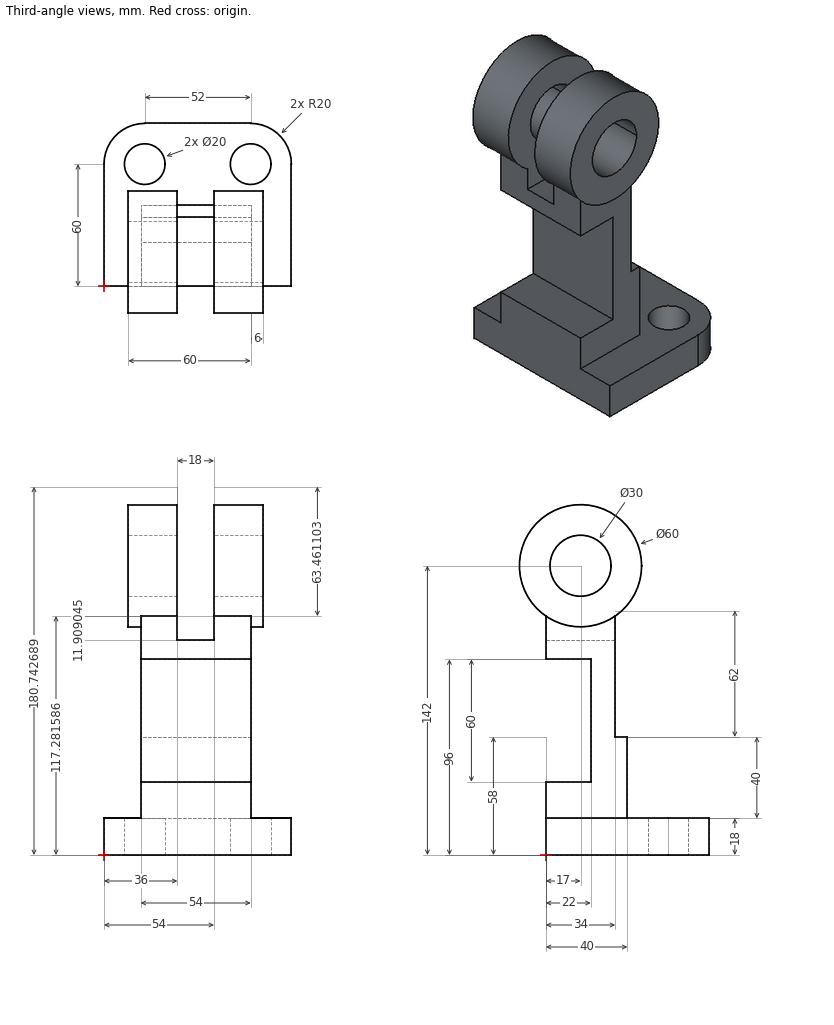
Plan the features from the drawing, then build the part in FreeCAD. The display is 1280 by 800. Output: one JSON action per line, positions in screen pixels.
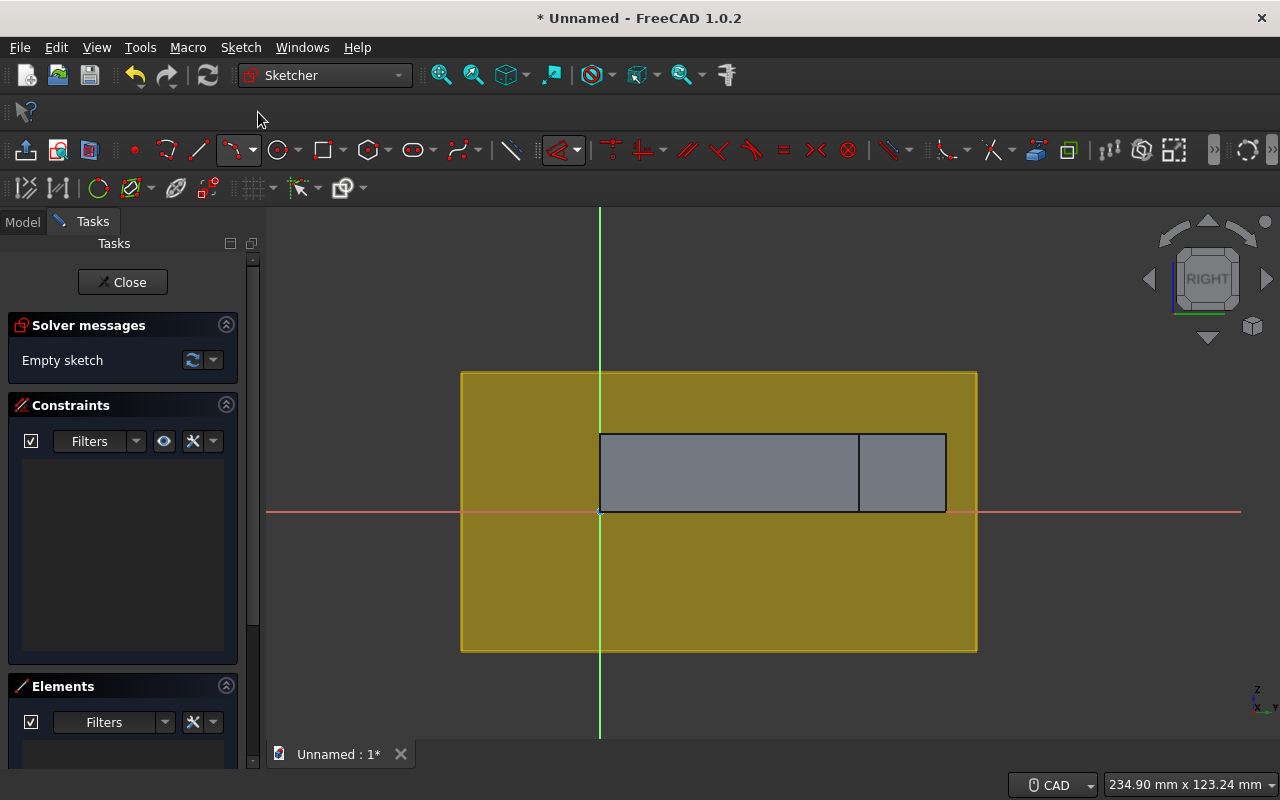
{"action": "left_click", "coordinate": [90, 150]}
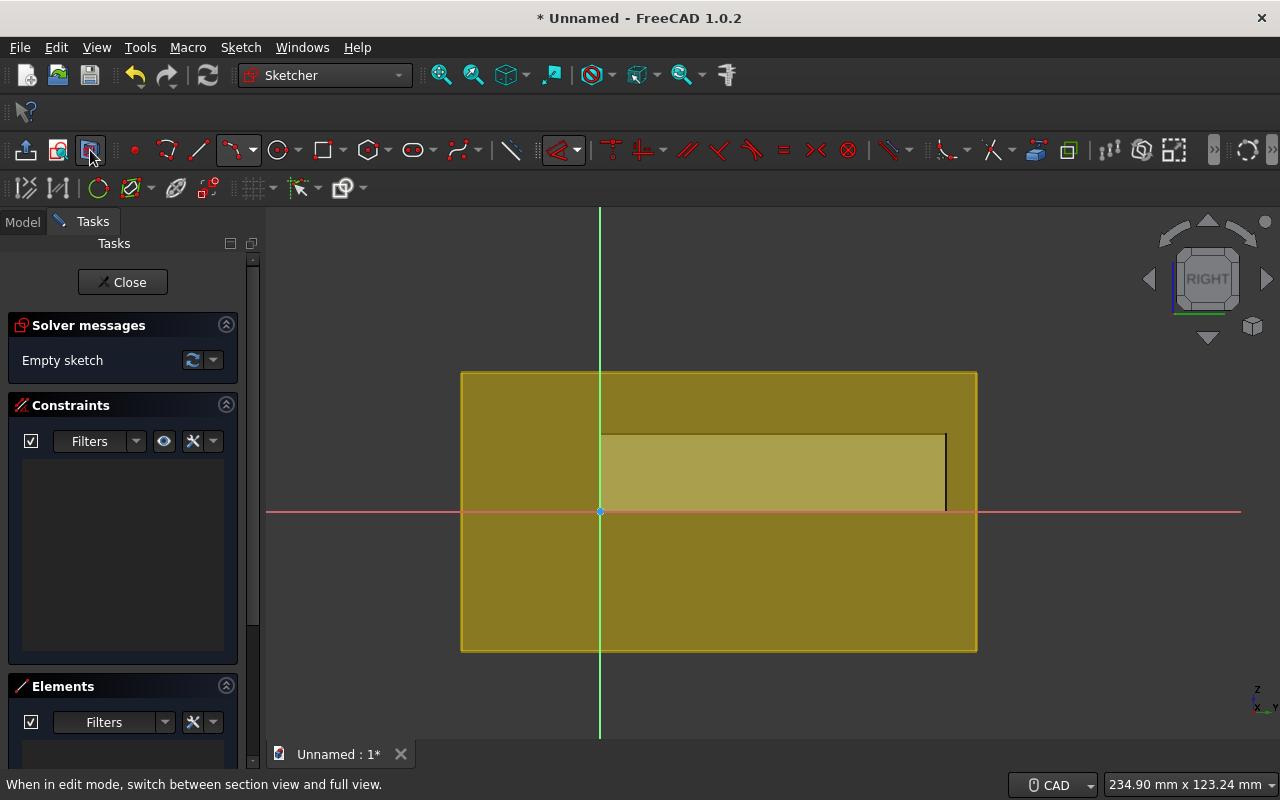
{"action": "left_click", "coordinate": [324, 150]}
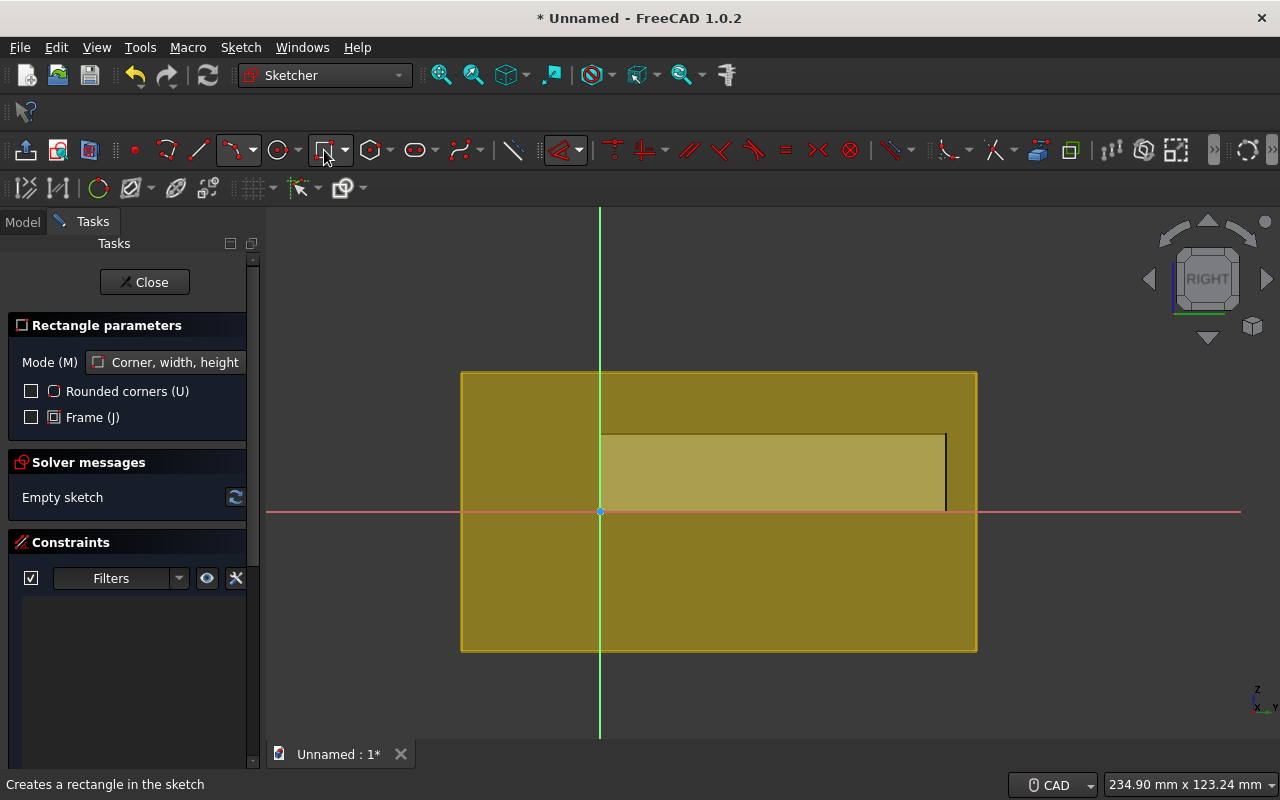
{"action": "left_click", "coordinate": [600, 261]}
{"action": "mouse_move", "coordinate": [773, 434]}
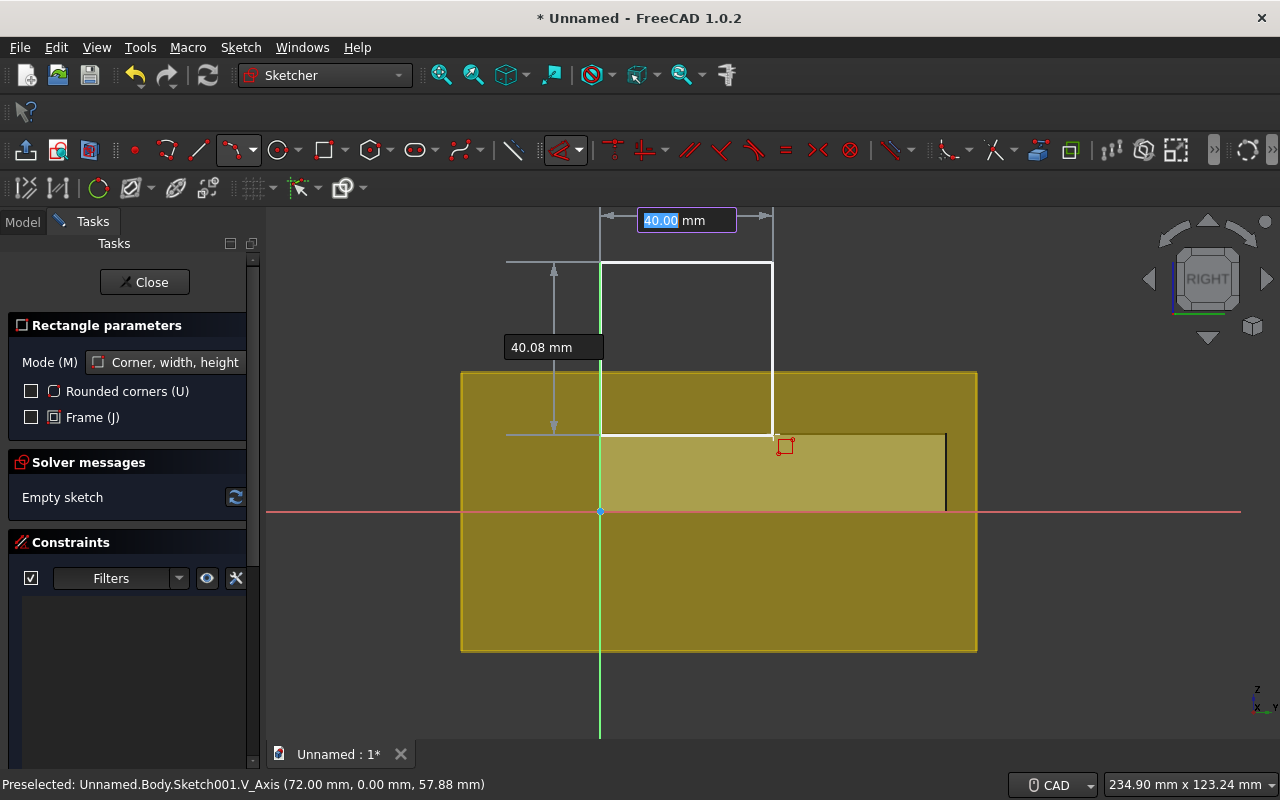
{"action": "type", "text": "40"}
{"action": "key", "text": "Tab"}
{"action": "type", "text": "40"}
{"action": "key", "text": "Return"}
{"action": "key", "text": "Escape"}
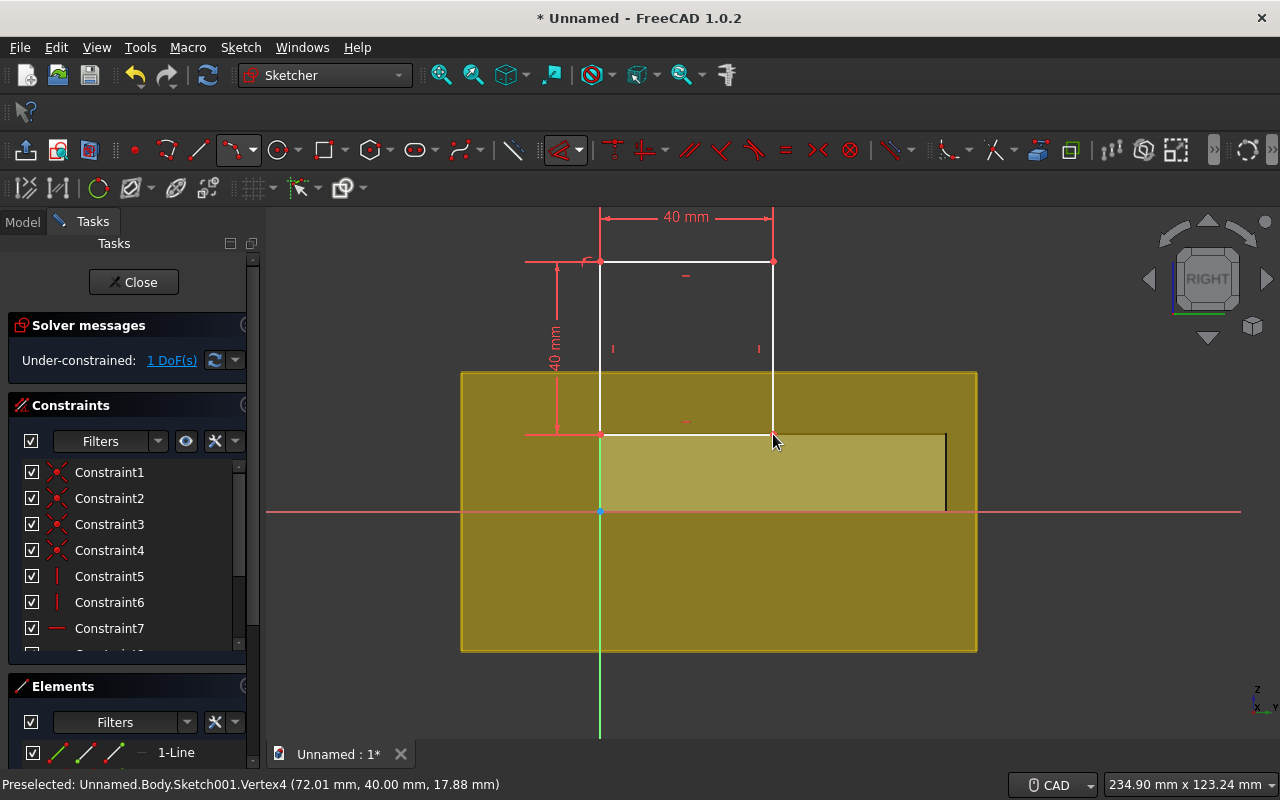
{"action": "left_click", "coordinate": [600, 262]}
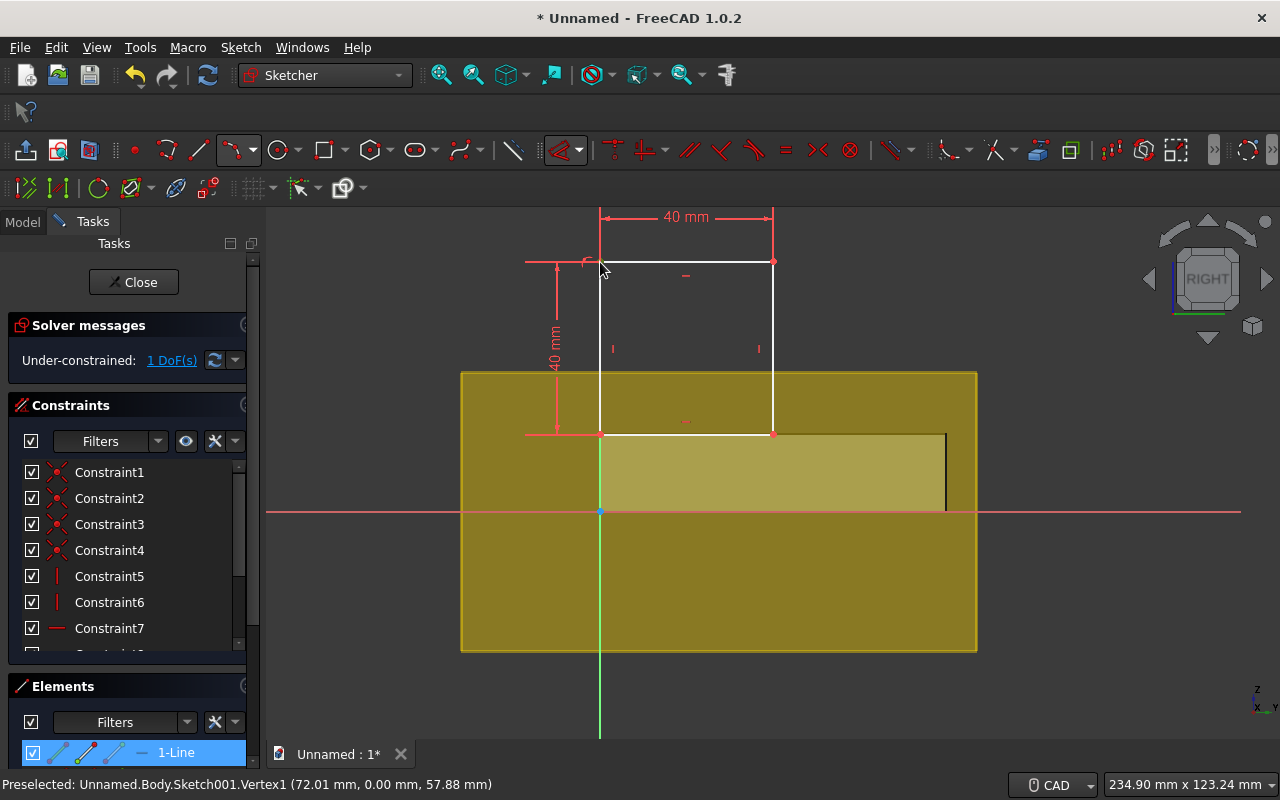
{"action": "left_click", "coordinate": [582, 150]}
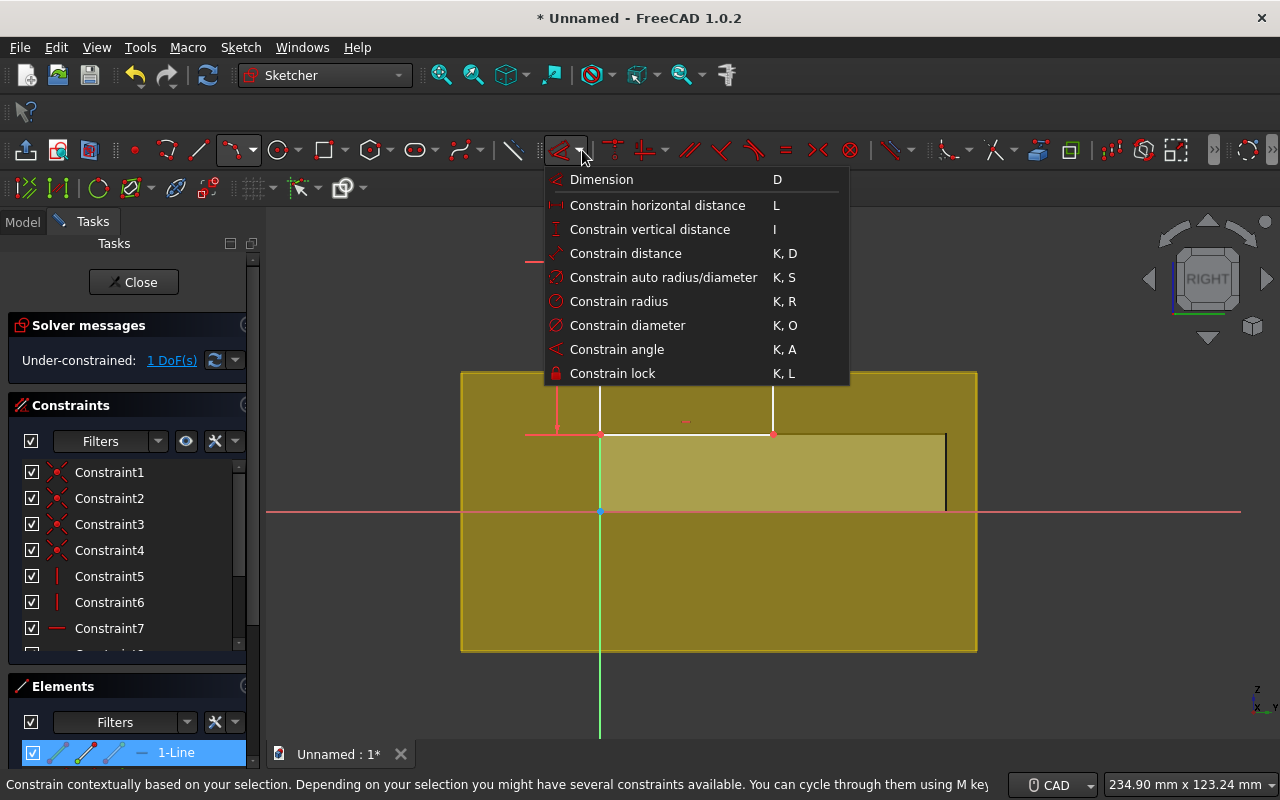
{"action": "left_click", "coordinate": [697, 229]}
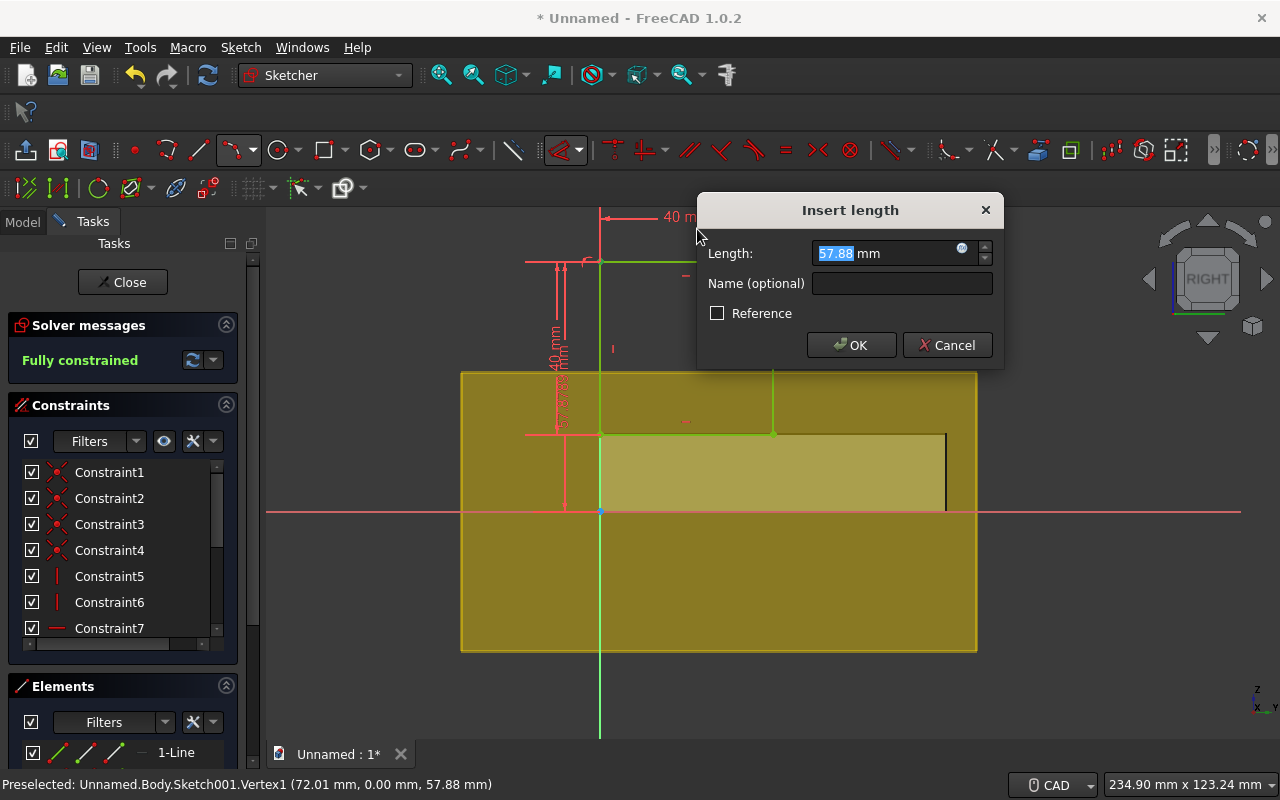
{"action": "type", "text": "58"}
{"action": "key", "text": "Return"}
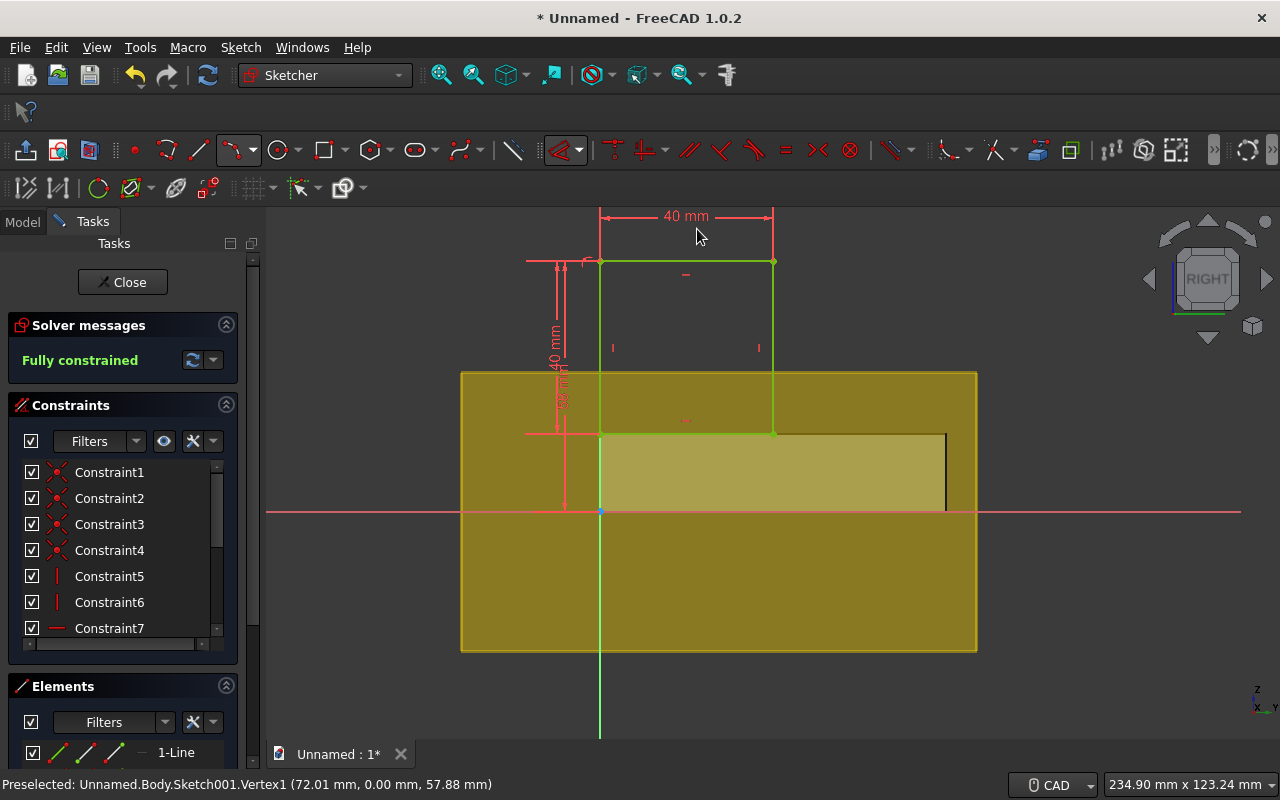
{"action": "left_click", "coordinate": [123, 282]}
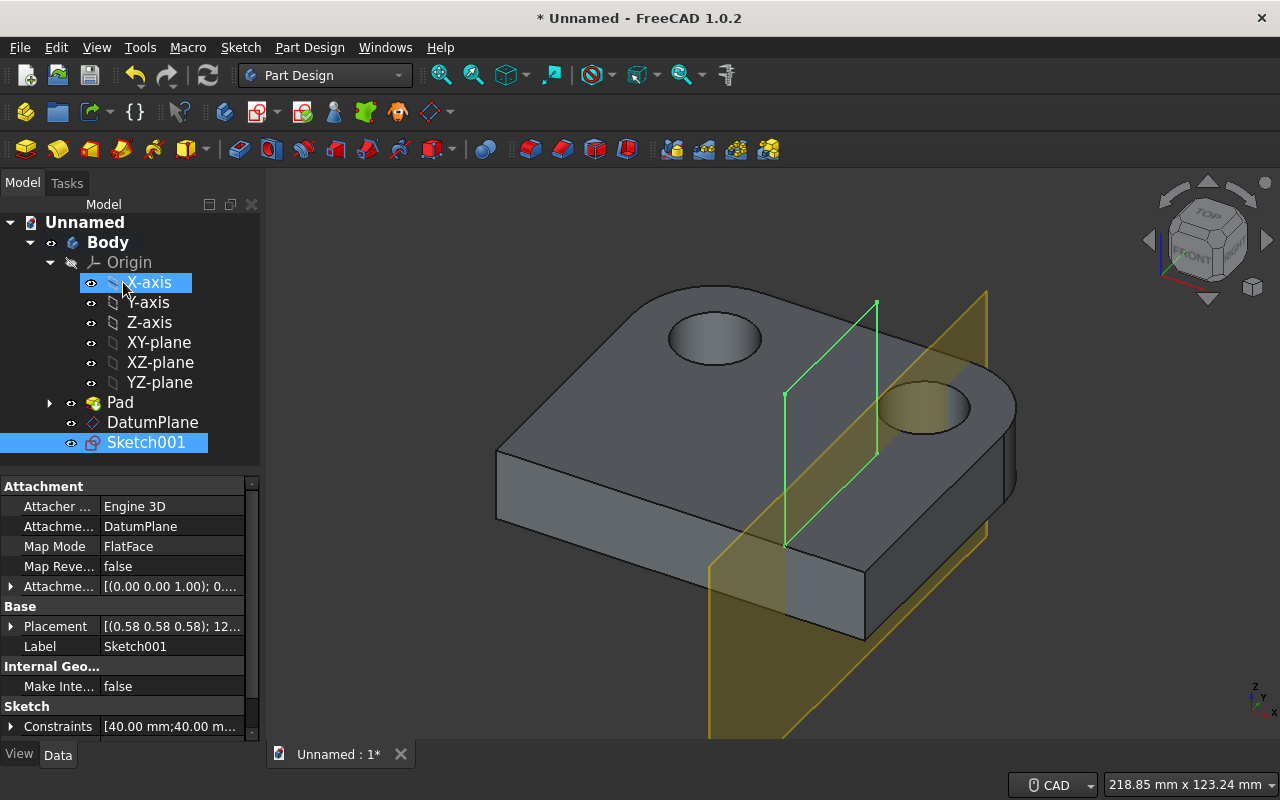
{"action": "left_click", "coordinate": [26, 150]}